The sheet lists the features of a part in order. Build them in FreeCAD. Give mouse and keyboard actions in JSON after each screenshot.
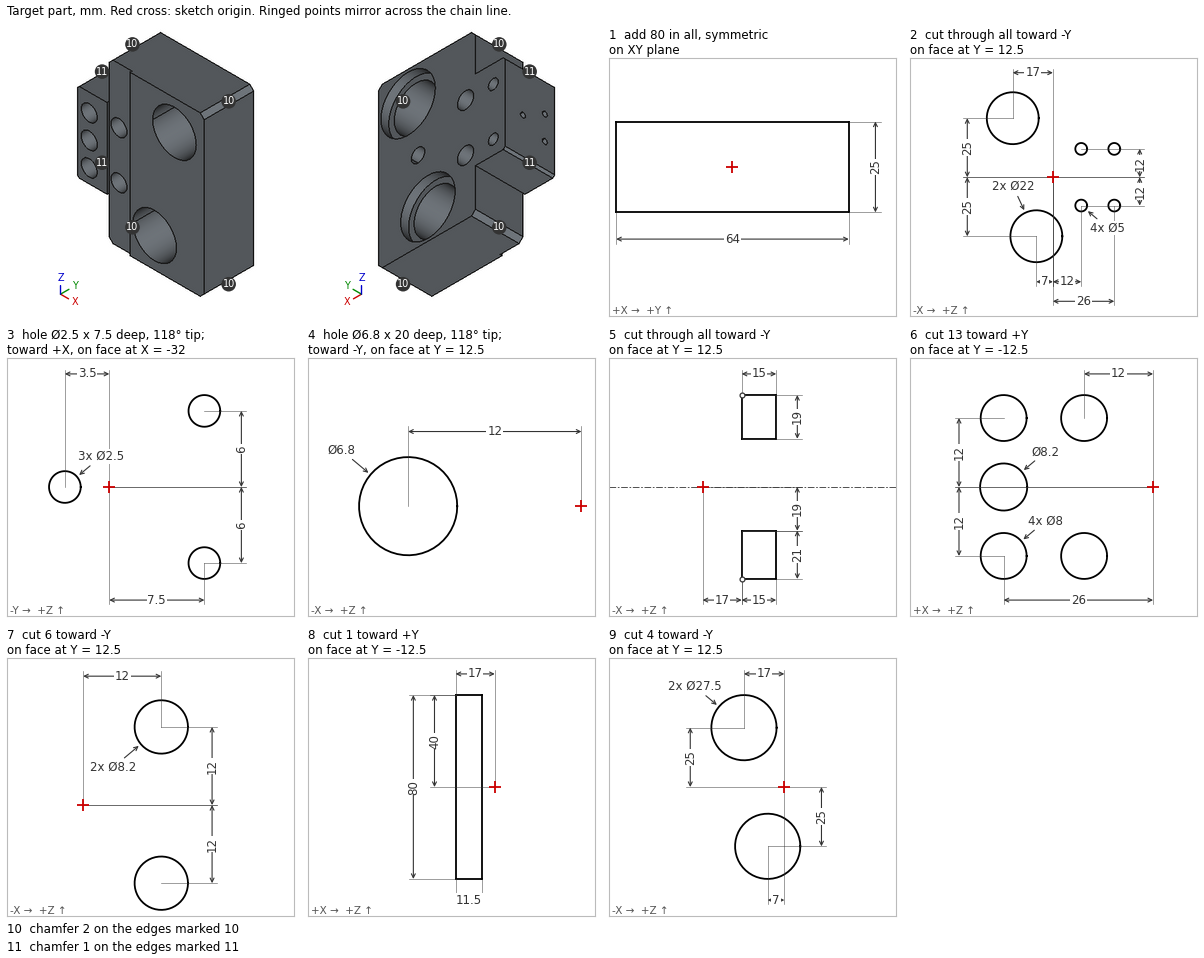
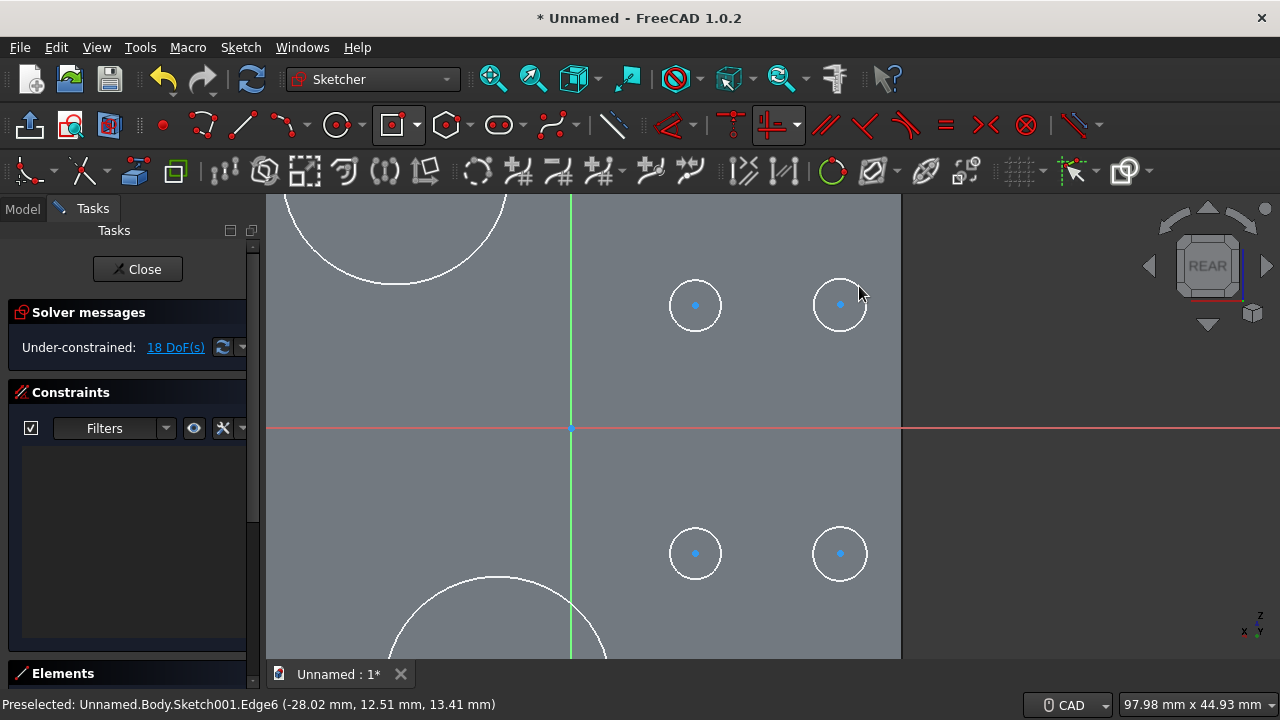
{"action": "left_click", "coordinate": [417, 610]}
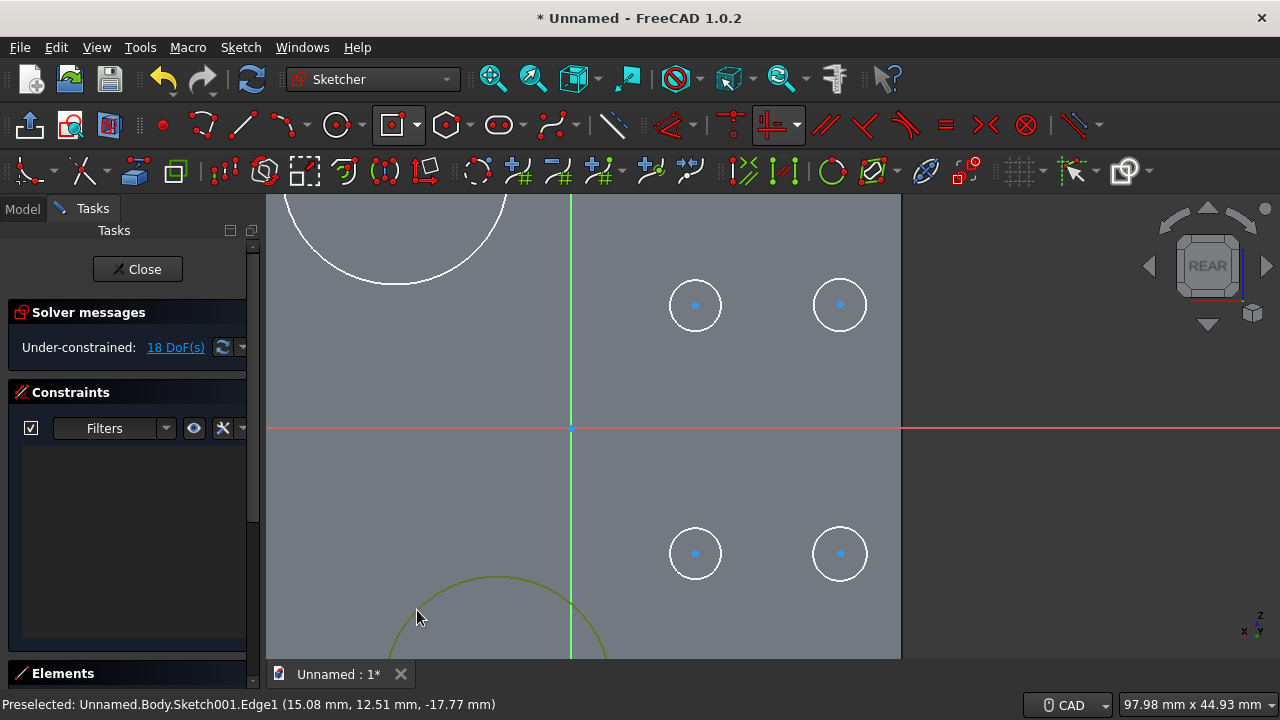
{"action": "left_click", "coordinate": [315, 252]}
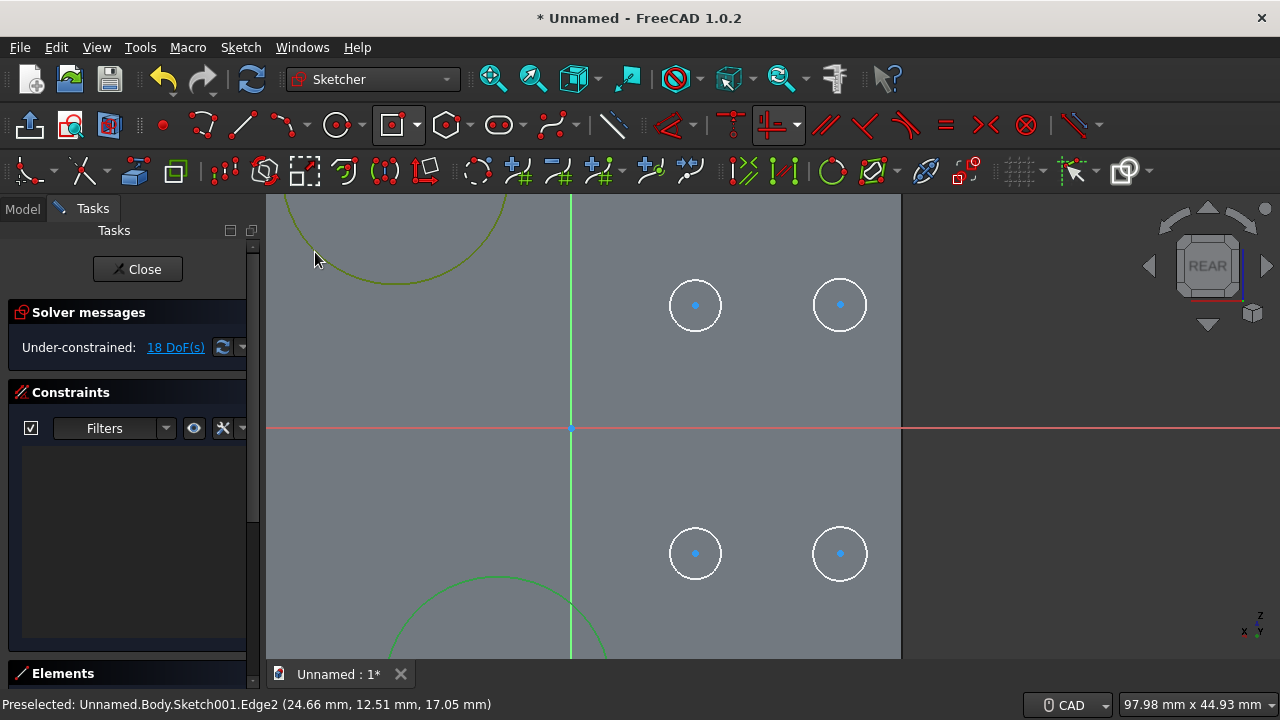
{"action": "left_click", "coordinate": [946, 126]}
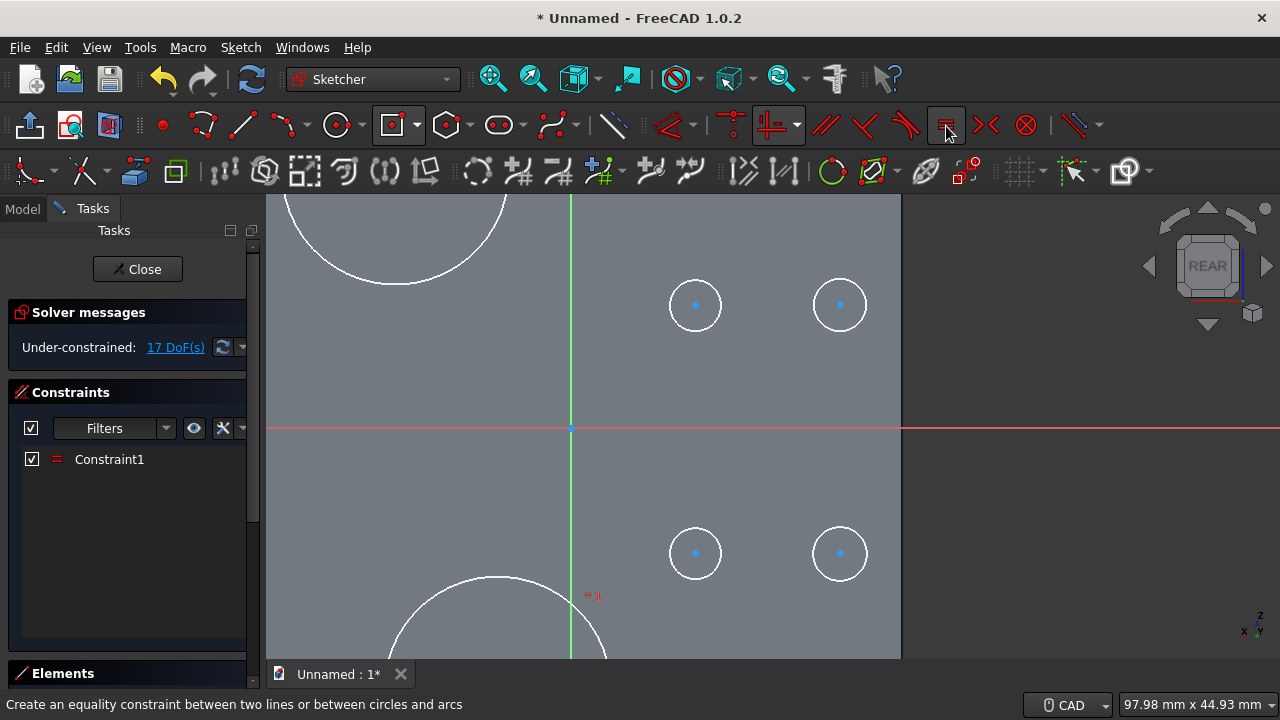
{"action": "left_click", "coordinate": [713, 536]}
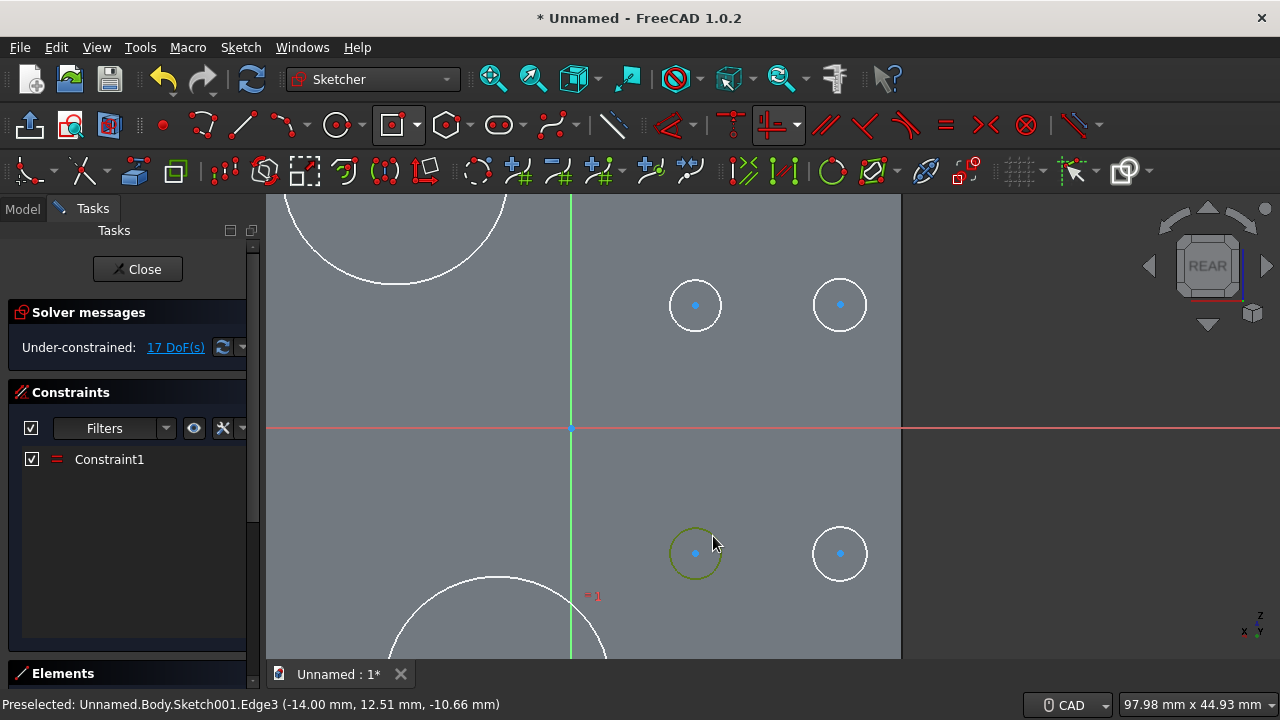
{"action": "left_click", "coordinate": [713, 288]}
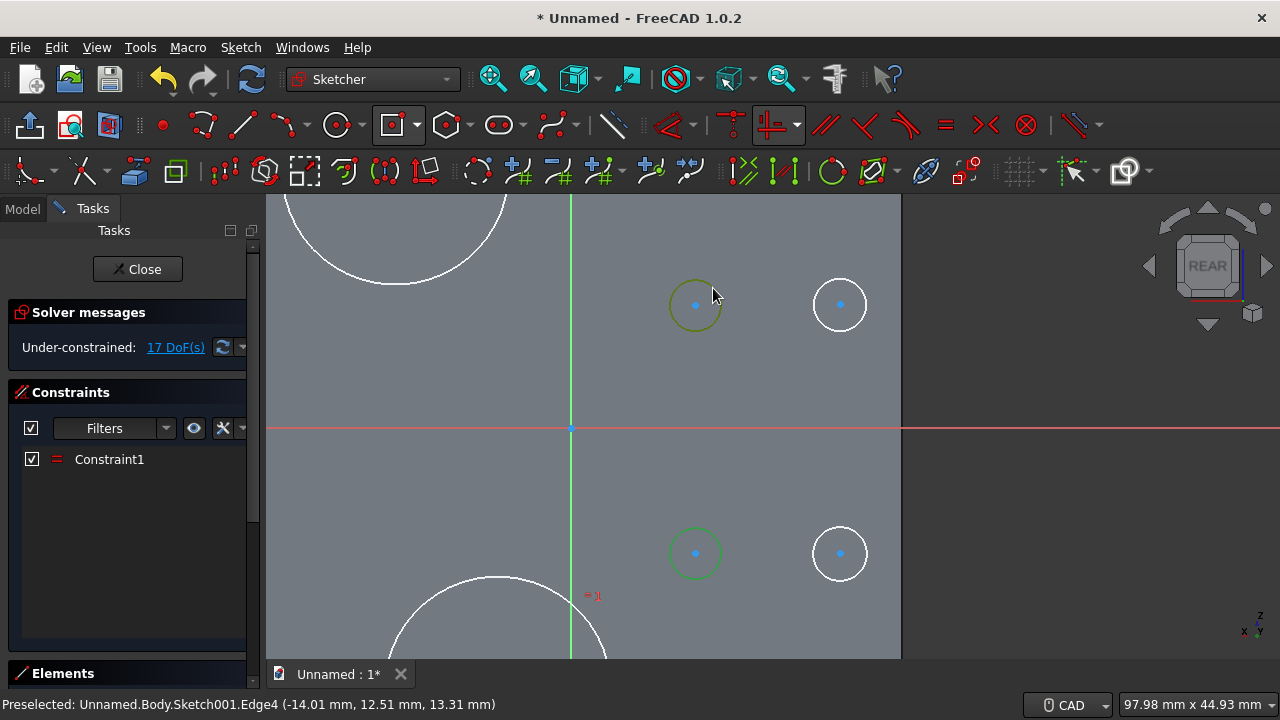
{"action": "left_click", "coordinate": [859, 535]}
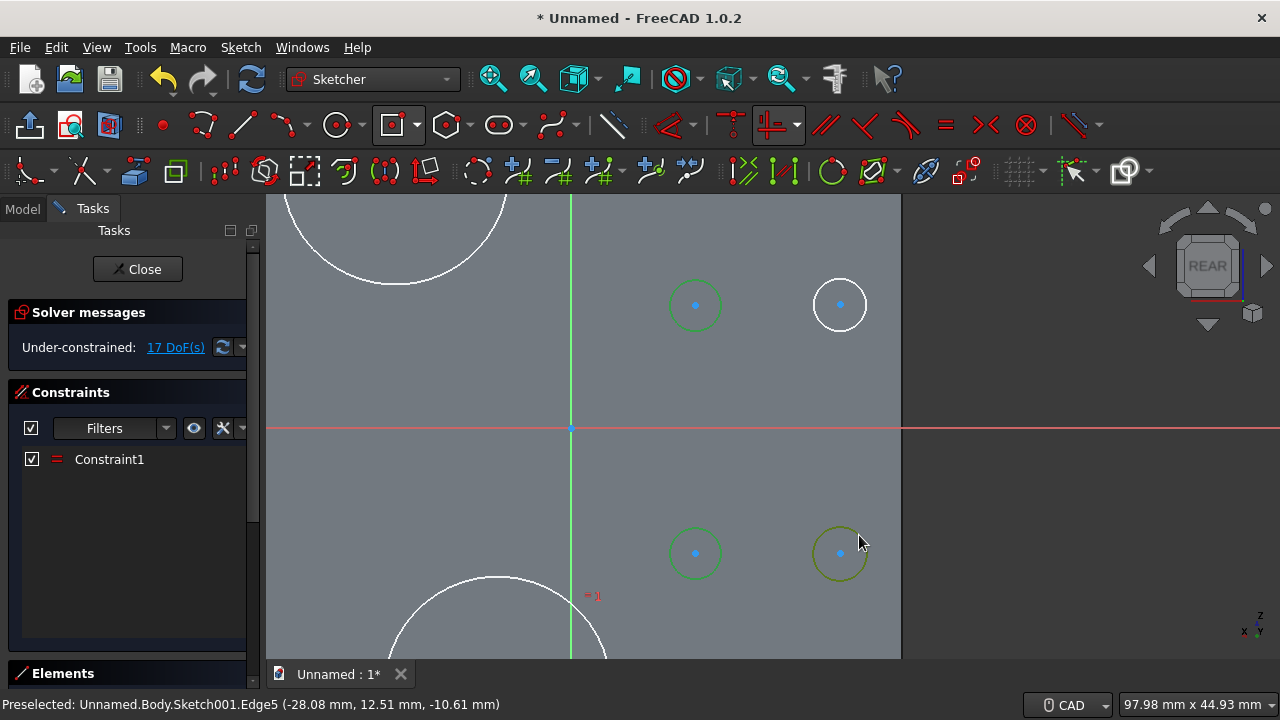
{"action": "left_click", "coordinate": [858, 286]}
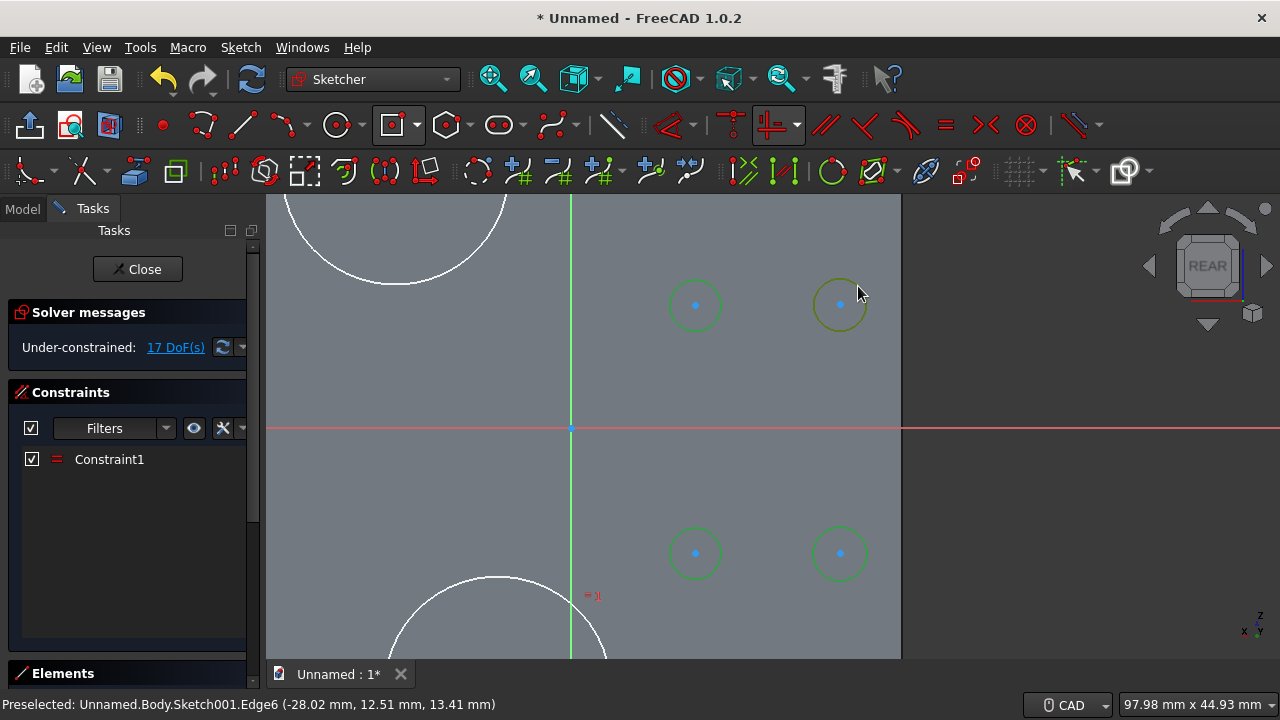
{"action": "left_click", "coordinate": [946, 126]}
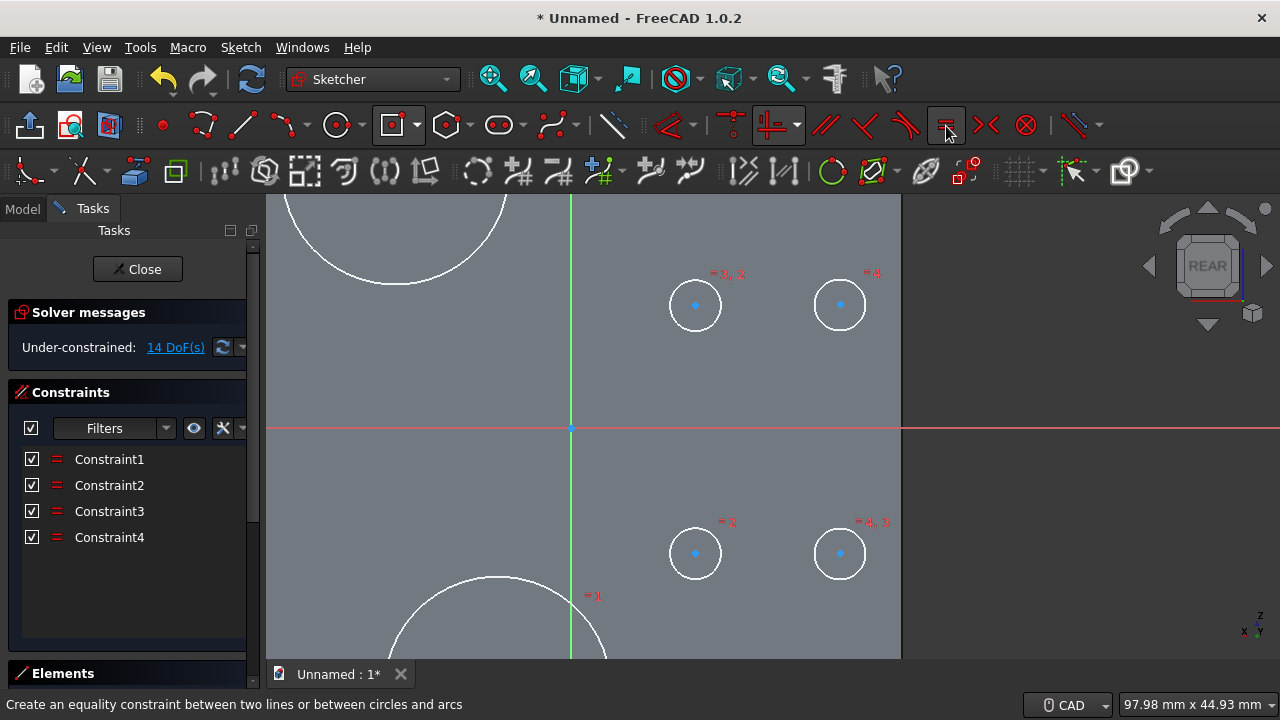
{"action": "left_click", "coordinate": [695, 554]}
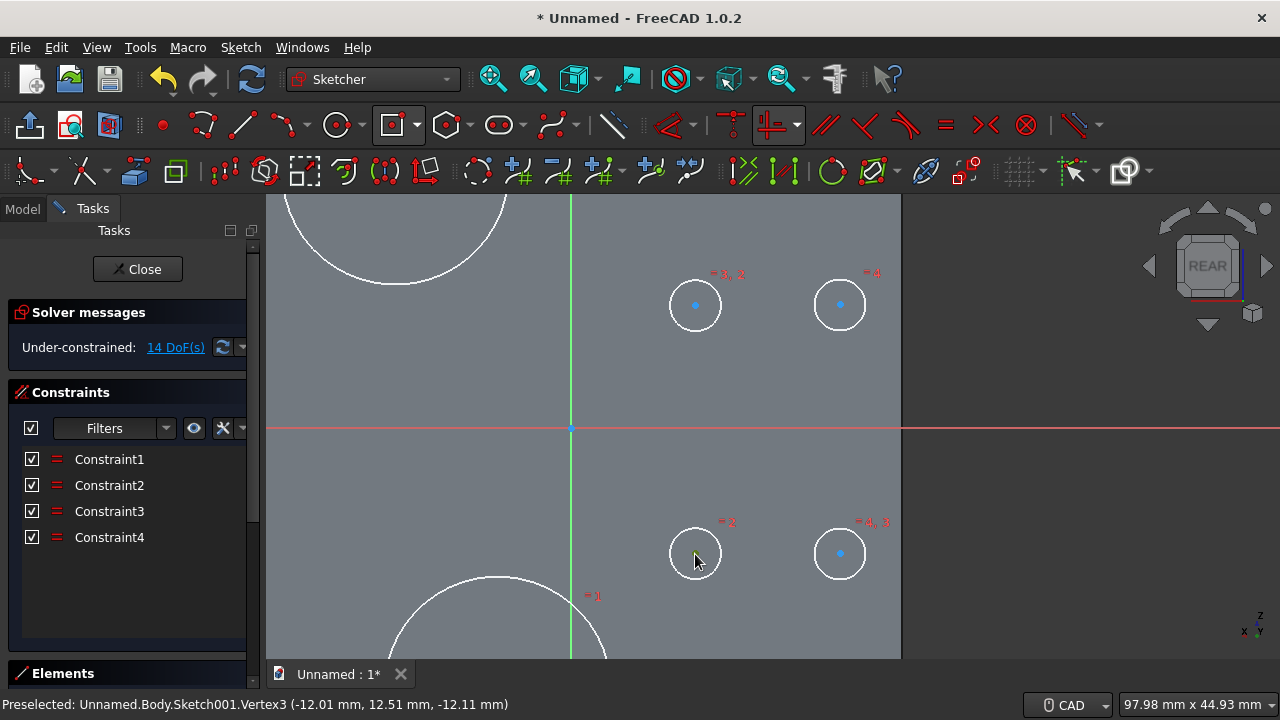
{"action": "left_click", "coordinate": [695, 306]}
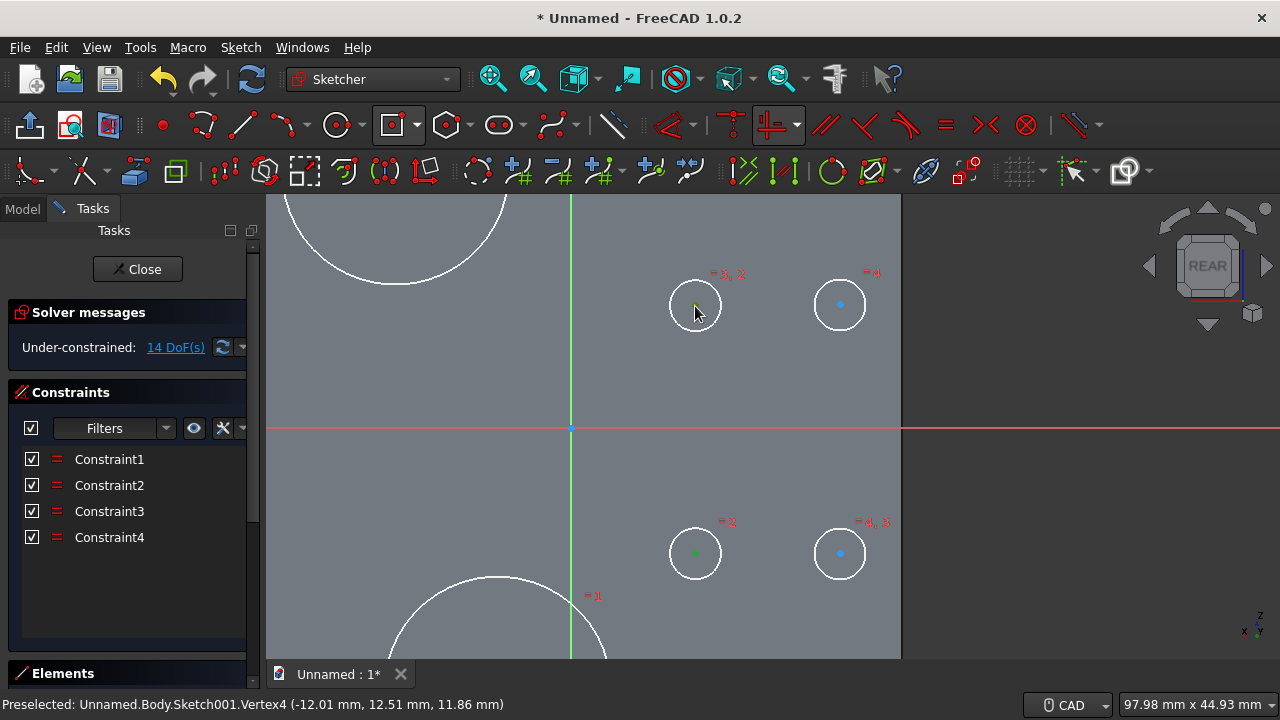
{"action": "key", "text": "v"}